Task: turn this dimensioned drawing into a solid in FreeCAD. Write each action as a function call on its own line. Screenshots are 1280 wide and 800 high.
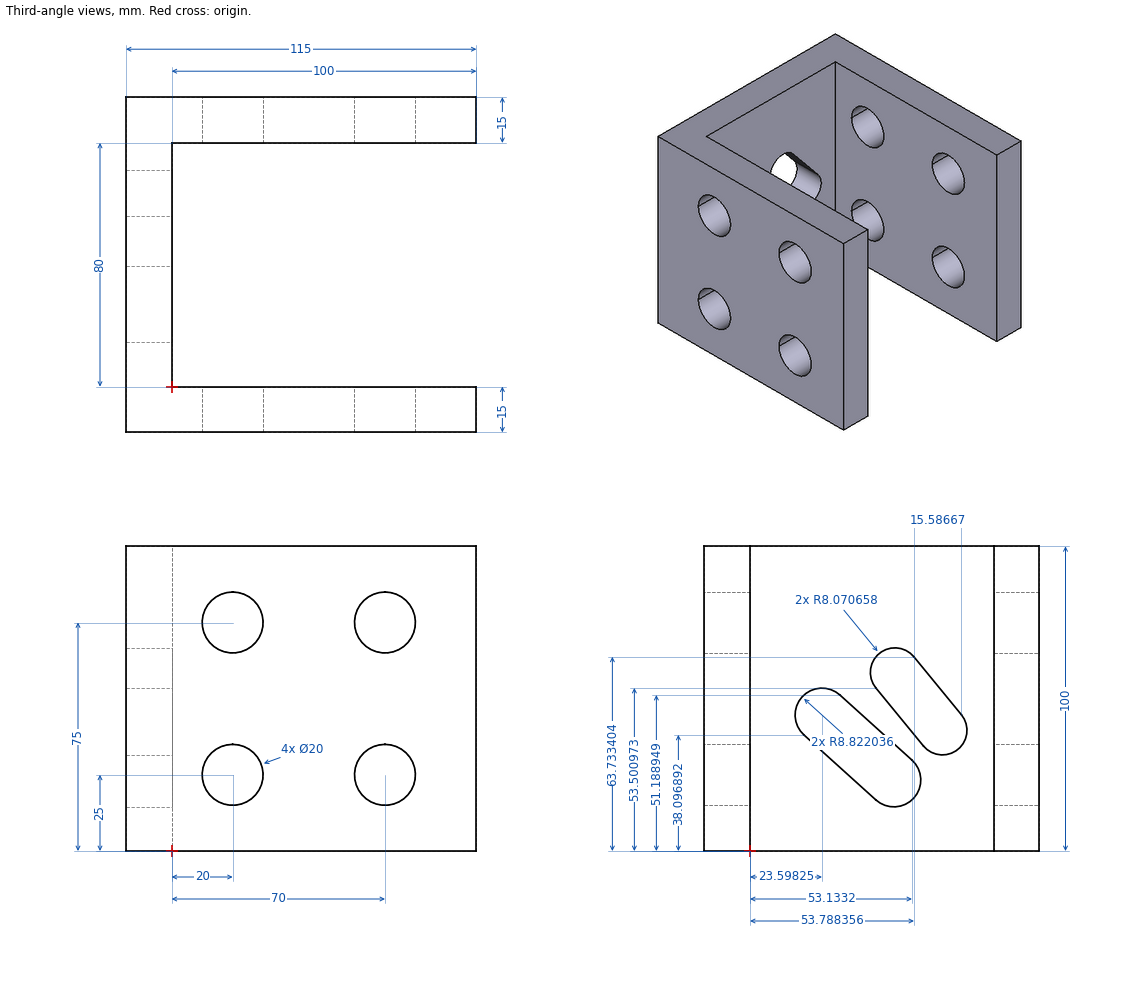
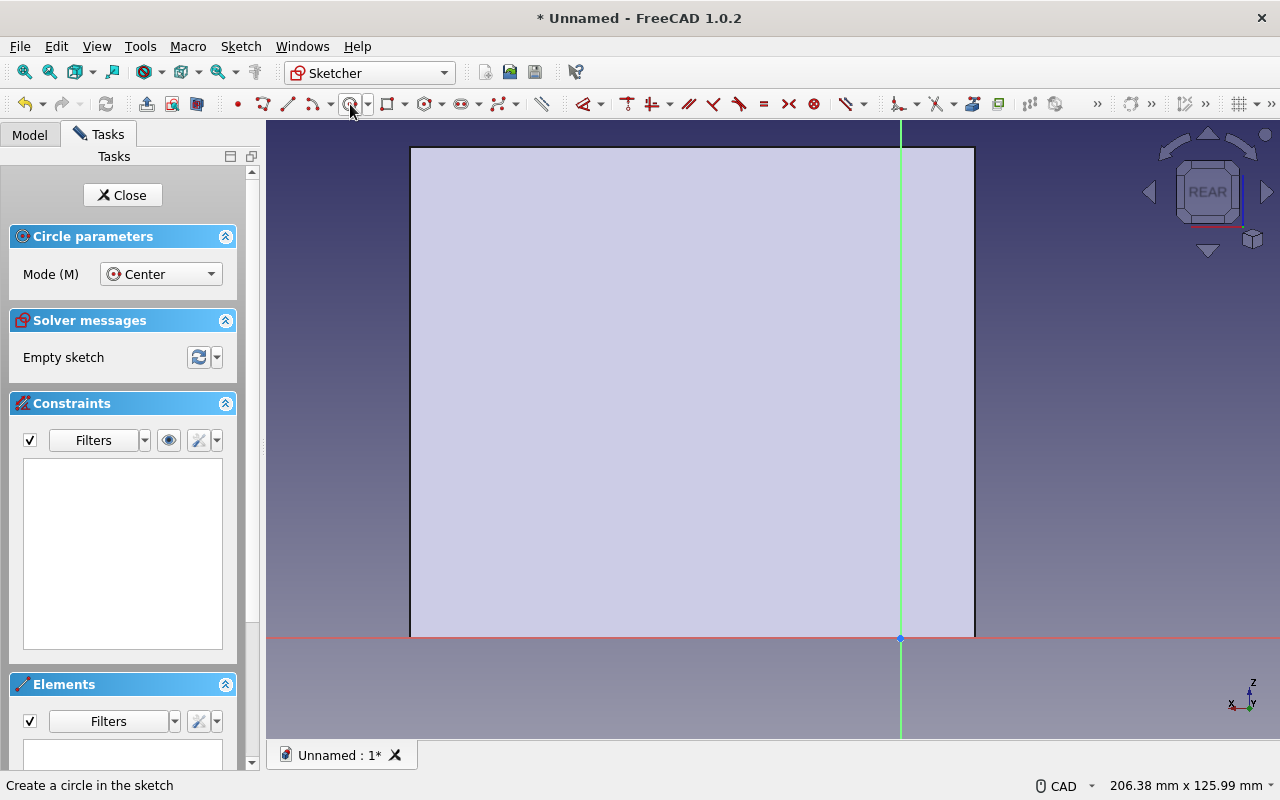
click(803, 515)
move(837, 481)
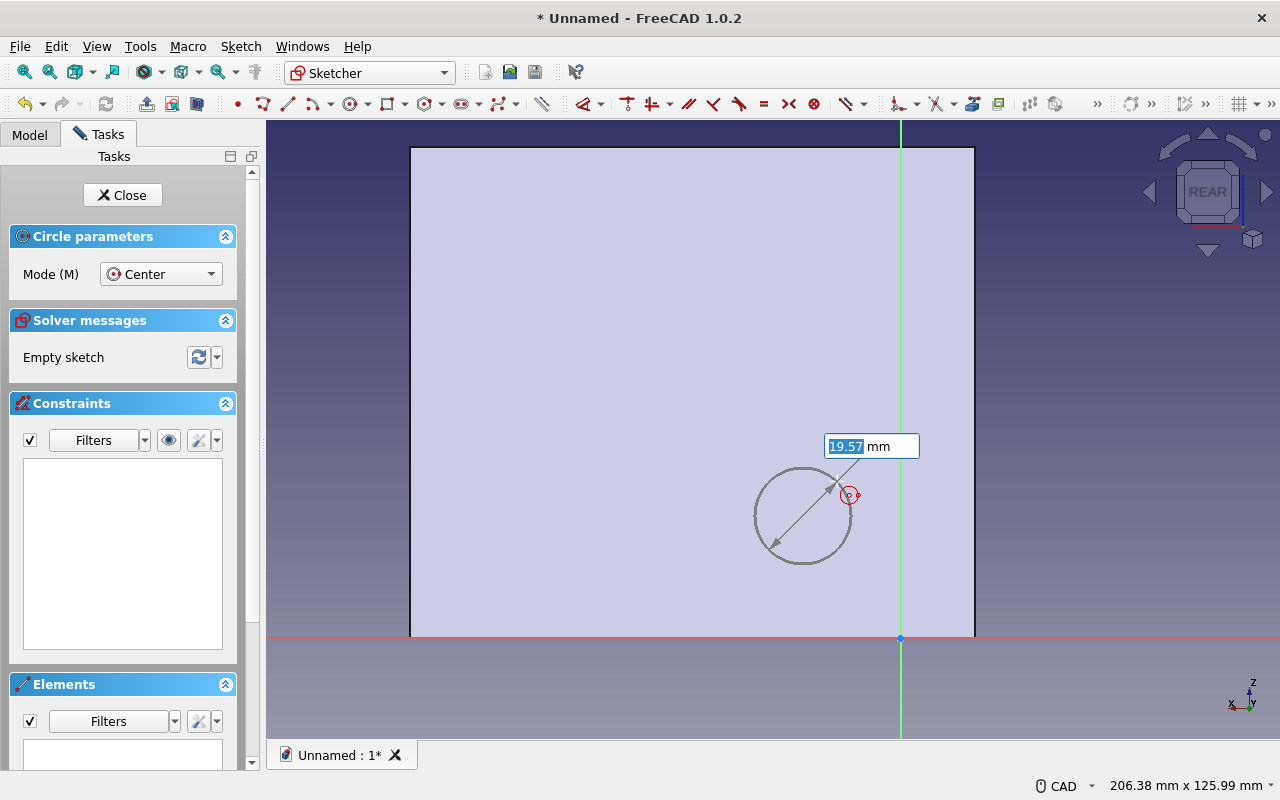
text(20)
key(Return)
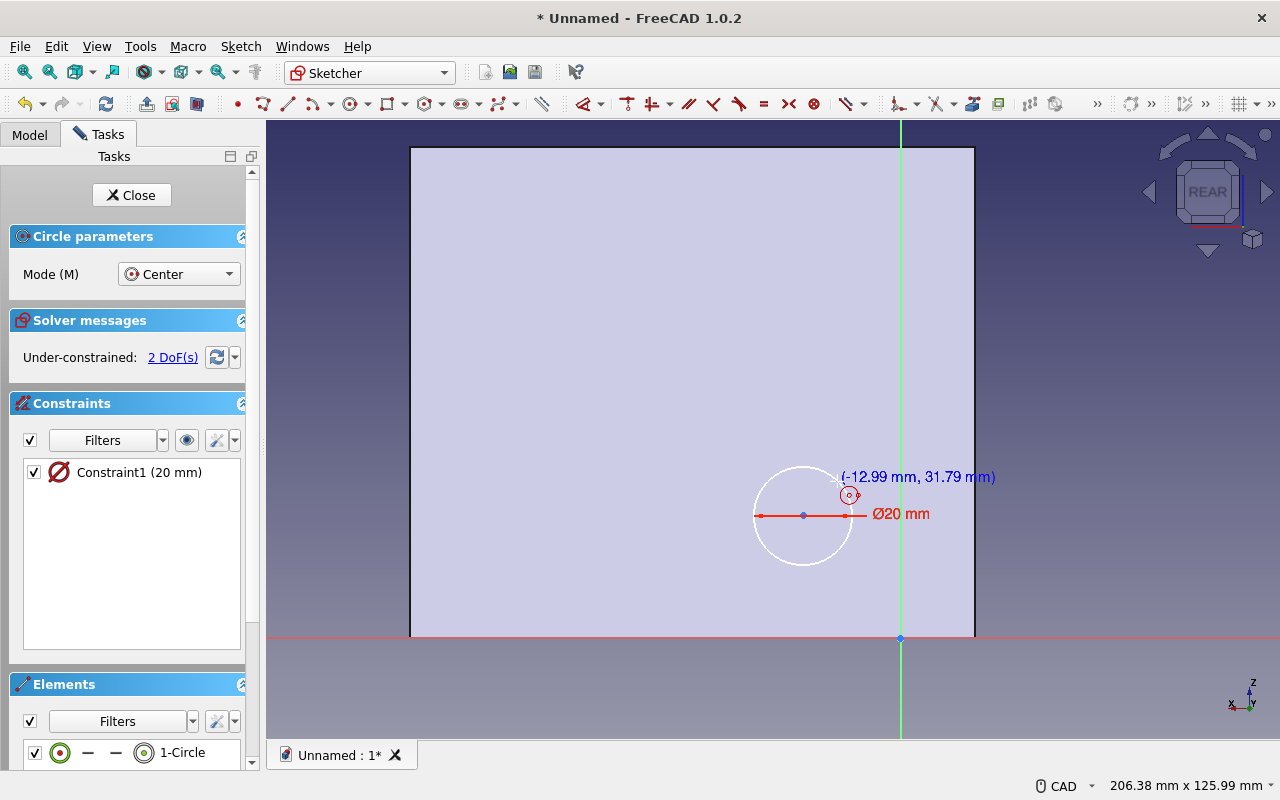
click(557, 515)
move(592, 481)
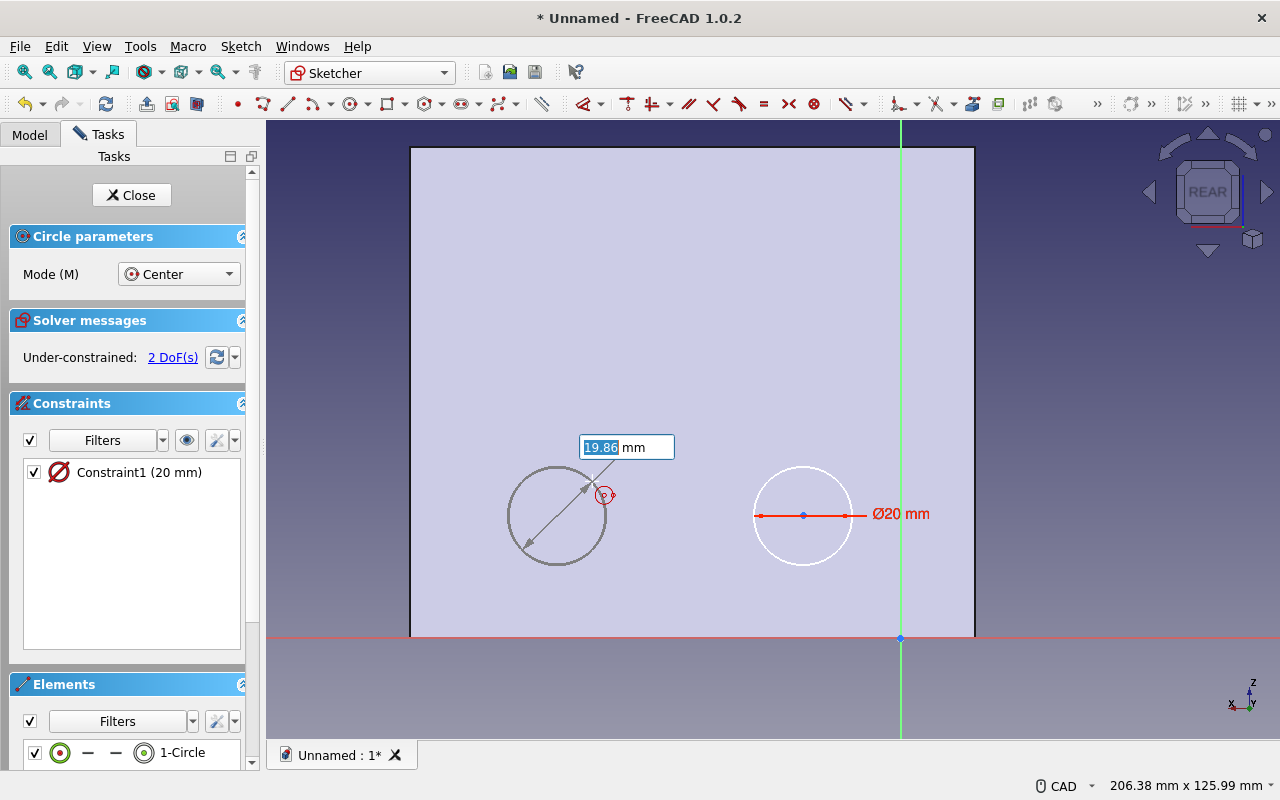
text(20)
key(Return)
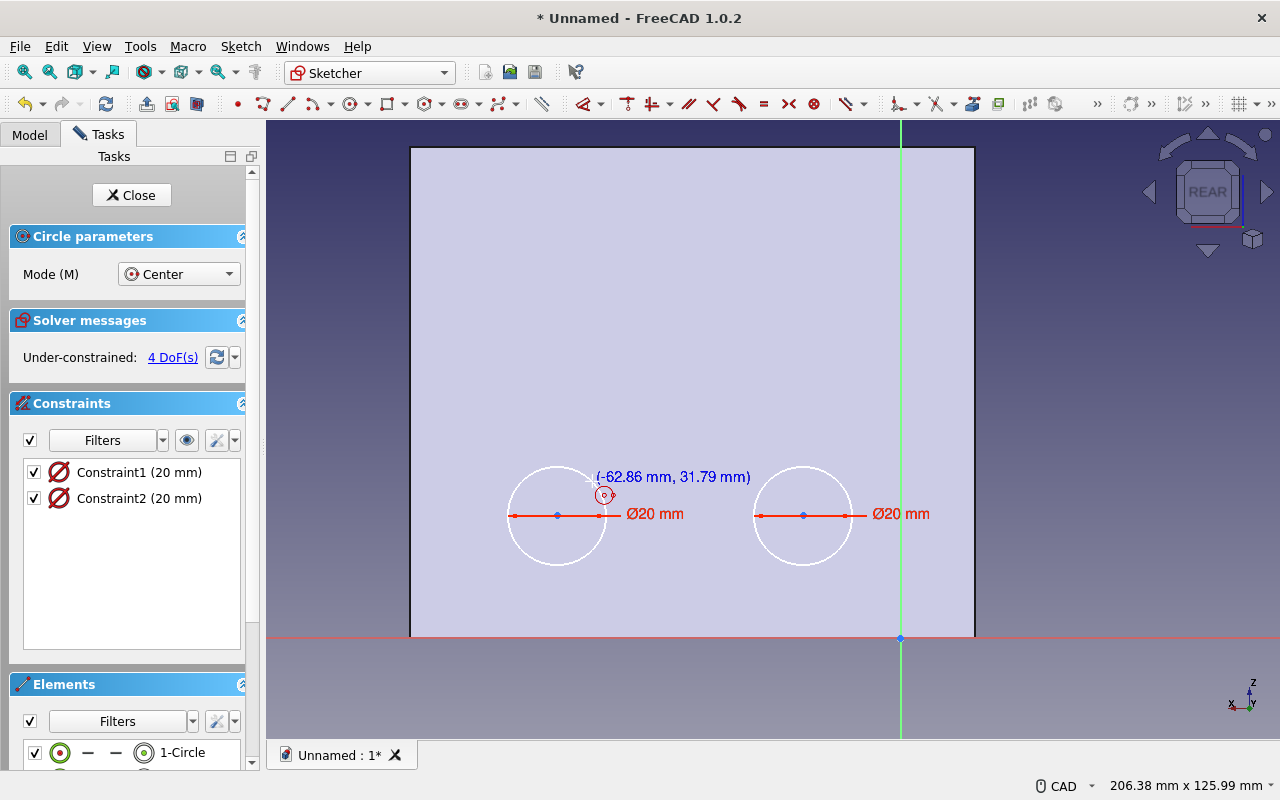
click(803, 270)
move(837, 235)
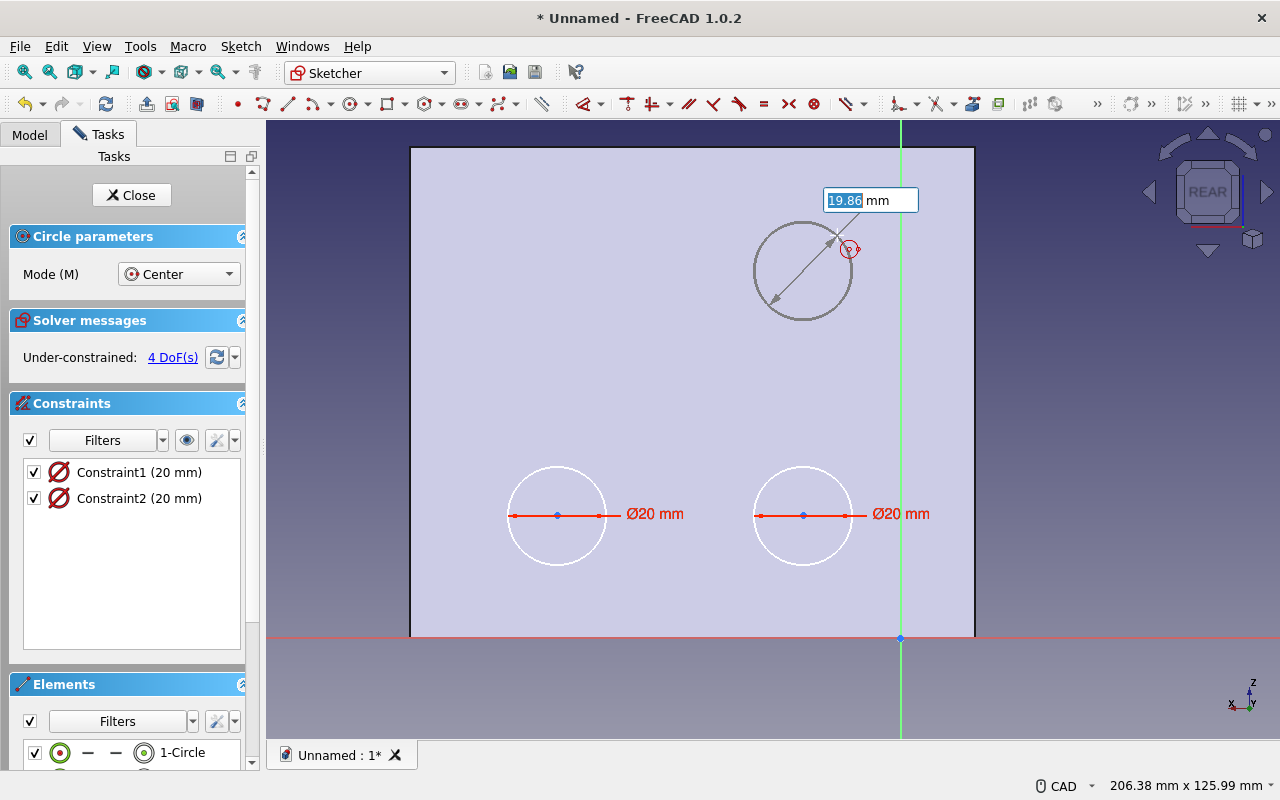
text(20)
key(Return)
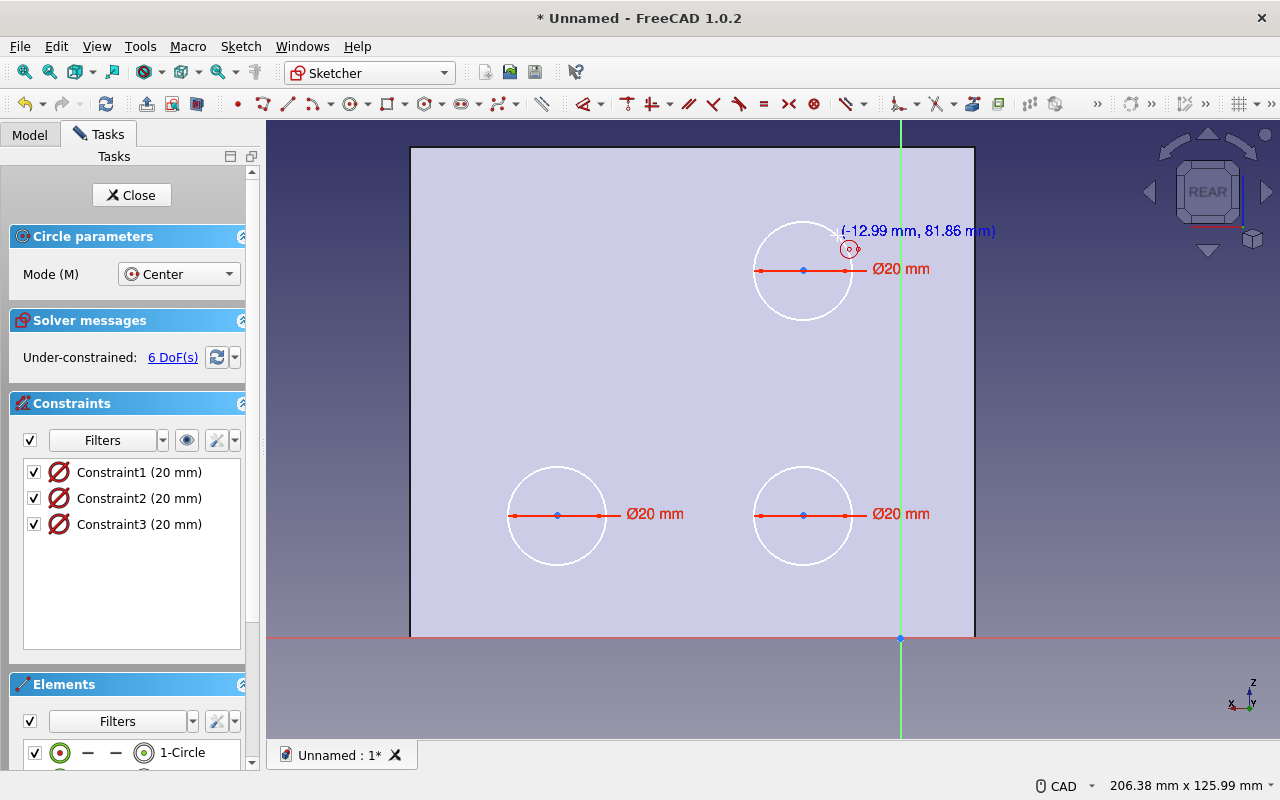
click(557, 270)
move(592, 235)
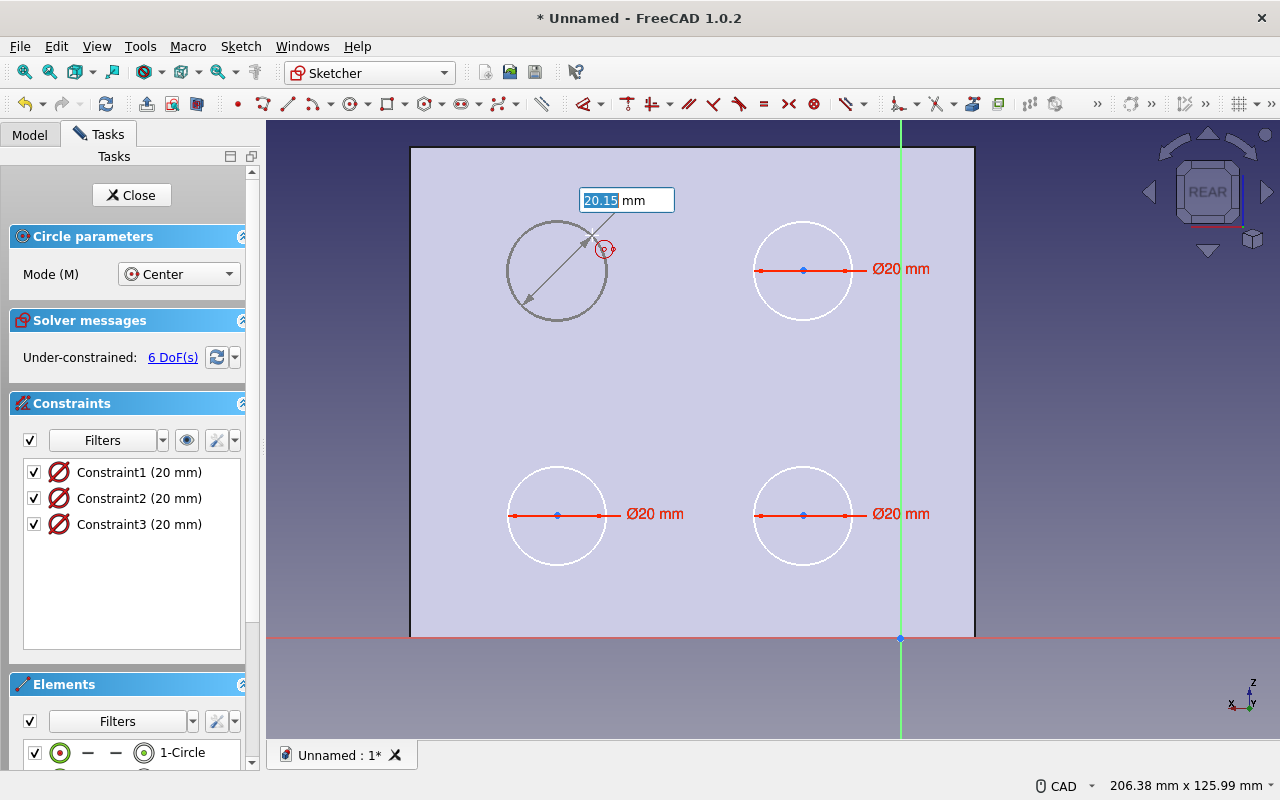
text(20)
key(Return)
key(Escape)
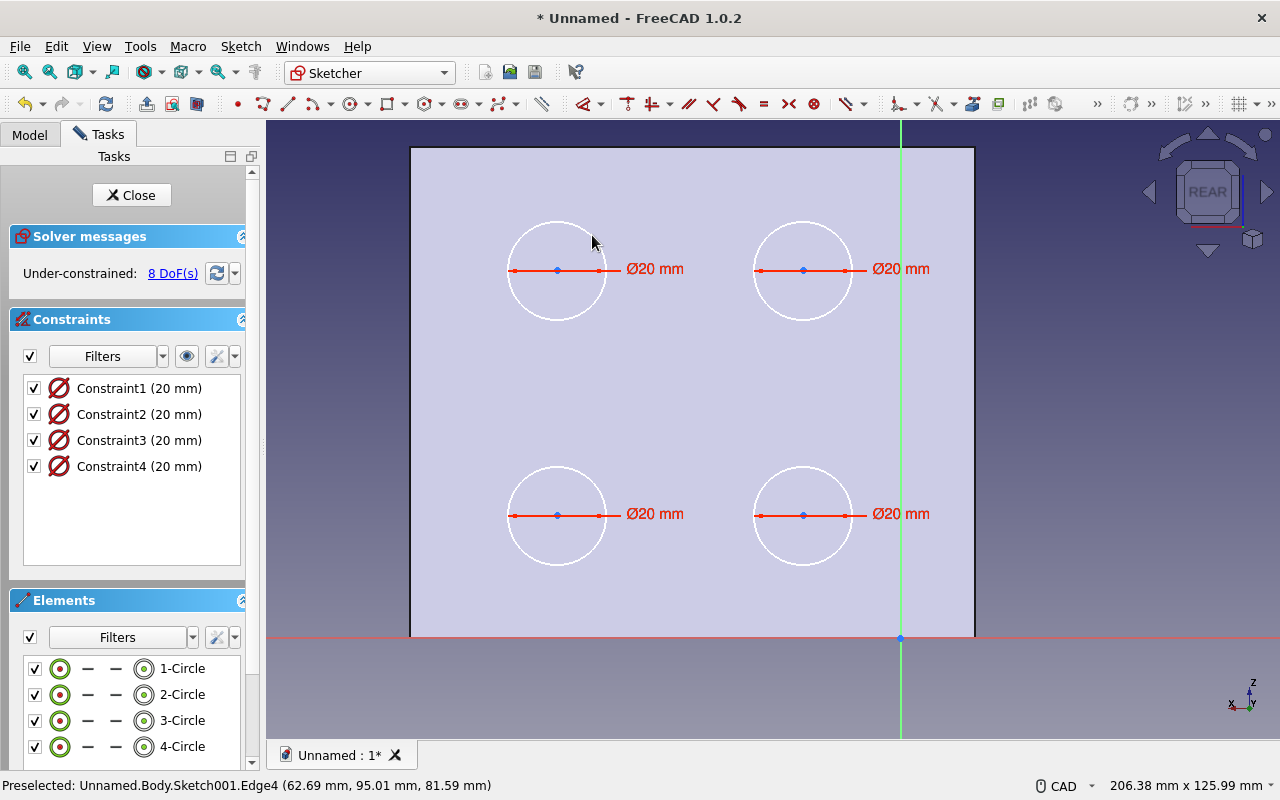
click(803, 516)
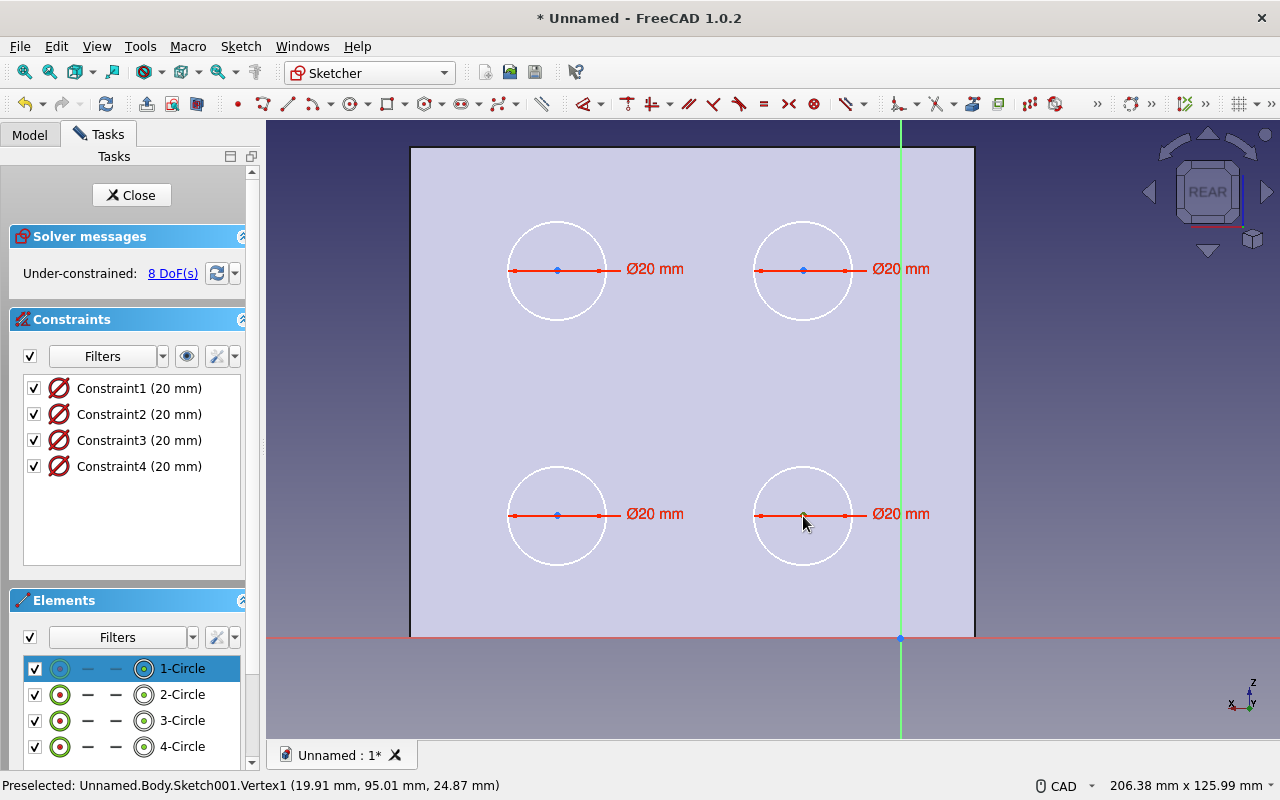
click(557, 516)